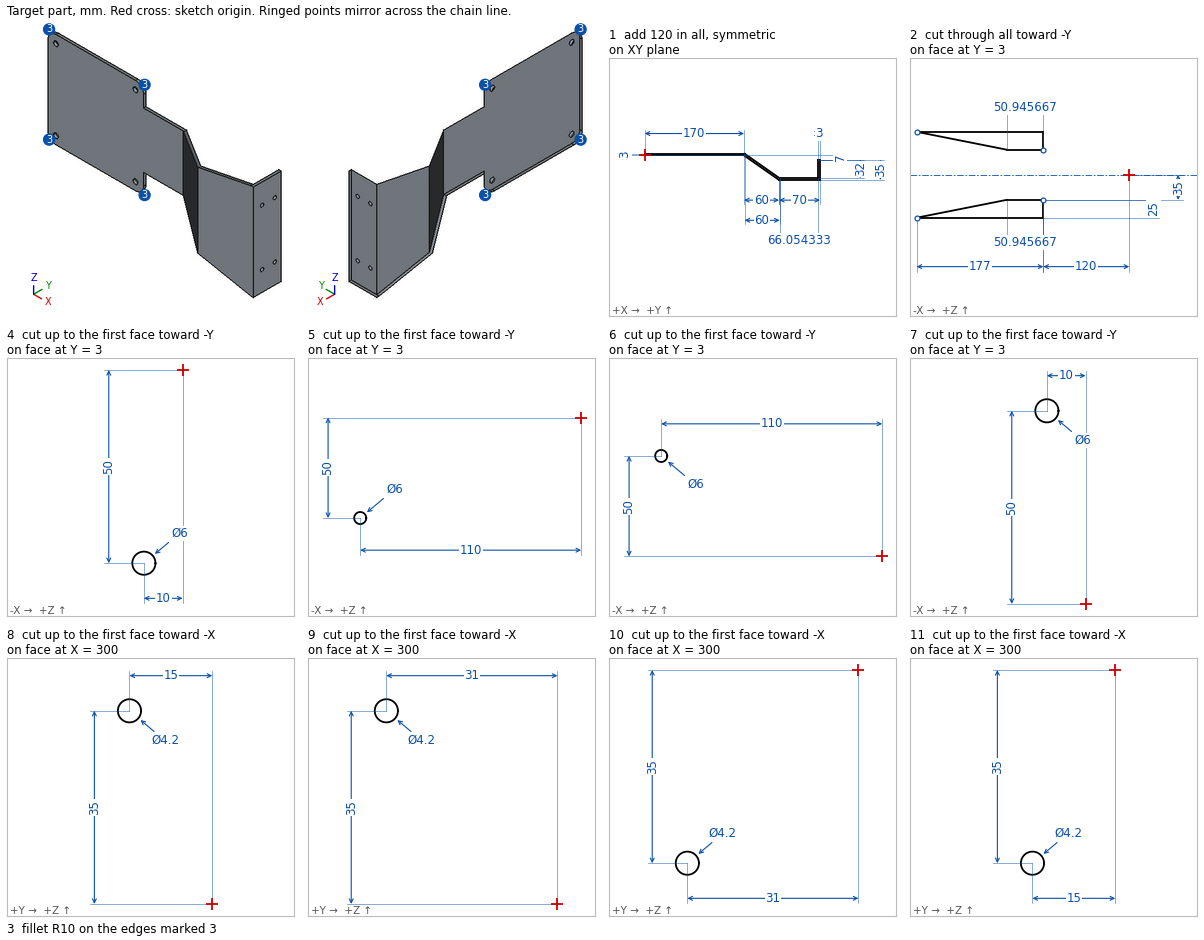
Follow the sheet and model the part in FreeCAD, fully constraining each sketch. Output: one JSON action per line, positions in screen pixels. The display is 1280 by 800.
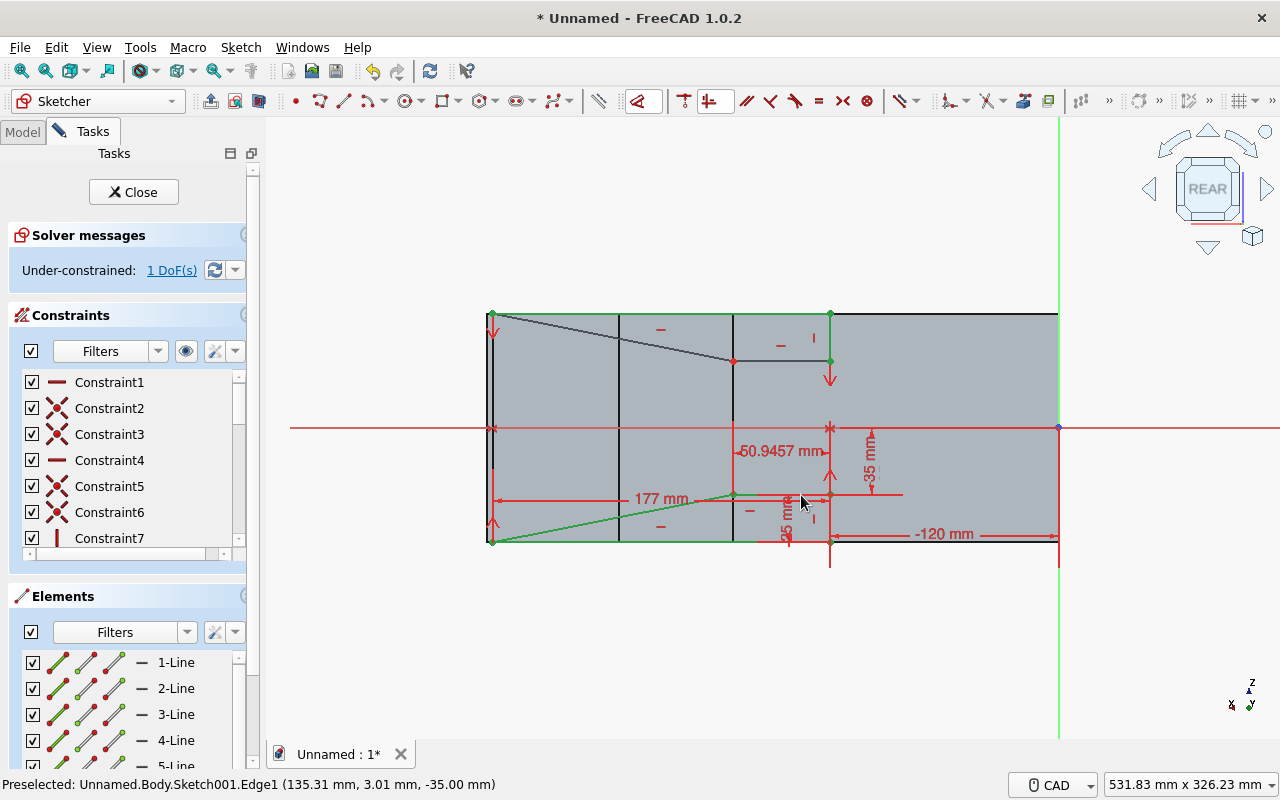
{"action": "left_click", "coordinate": [762, 361]}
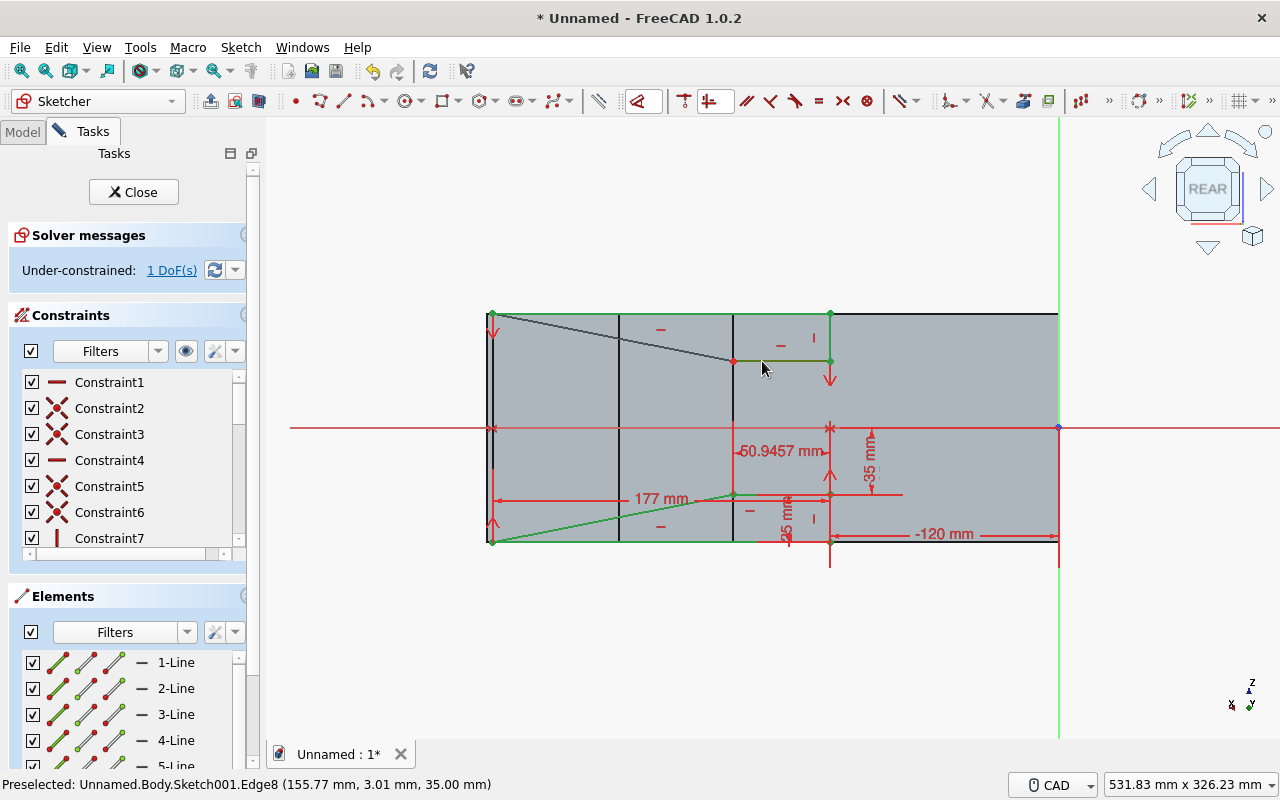
{"action": "key", "text": "l"}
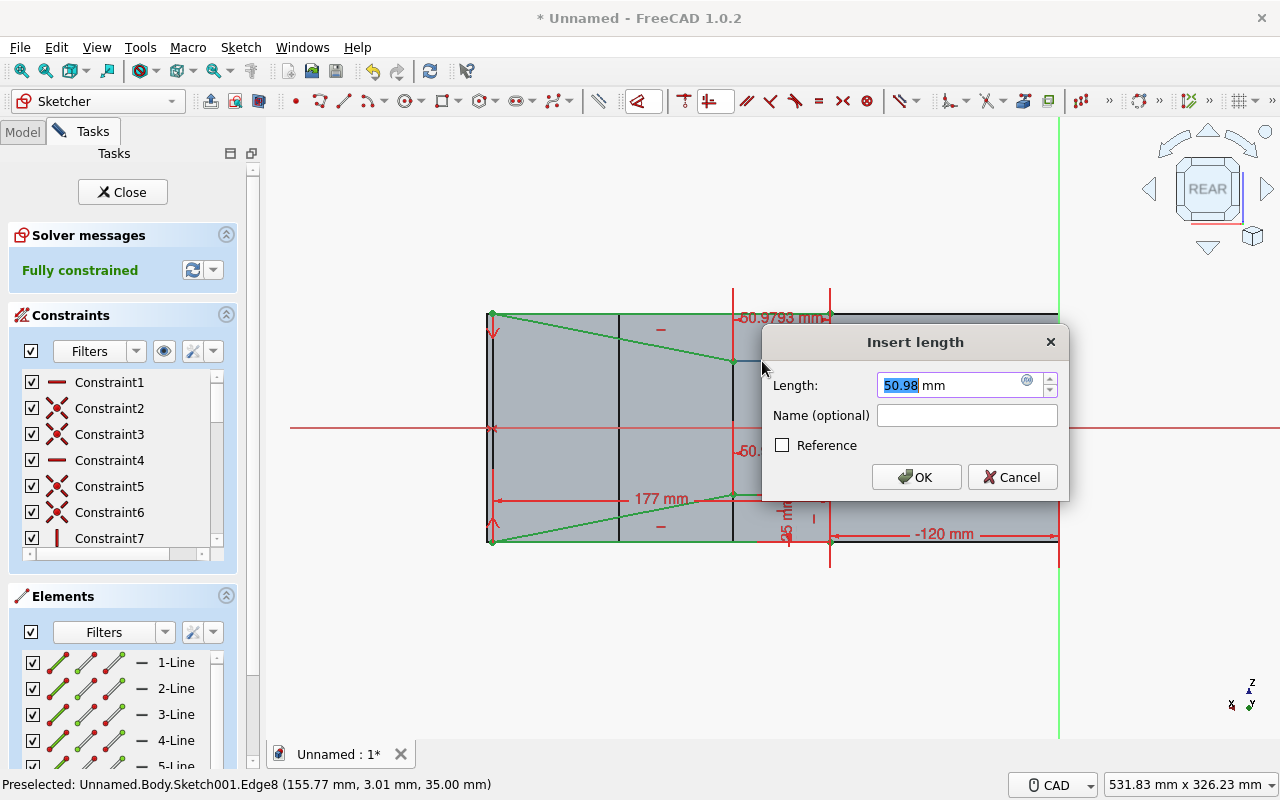
{"action": "type", "text": "50.945667"}
{"action": "key", "text": "Return"}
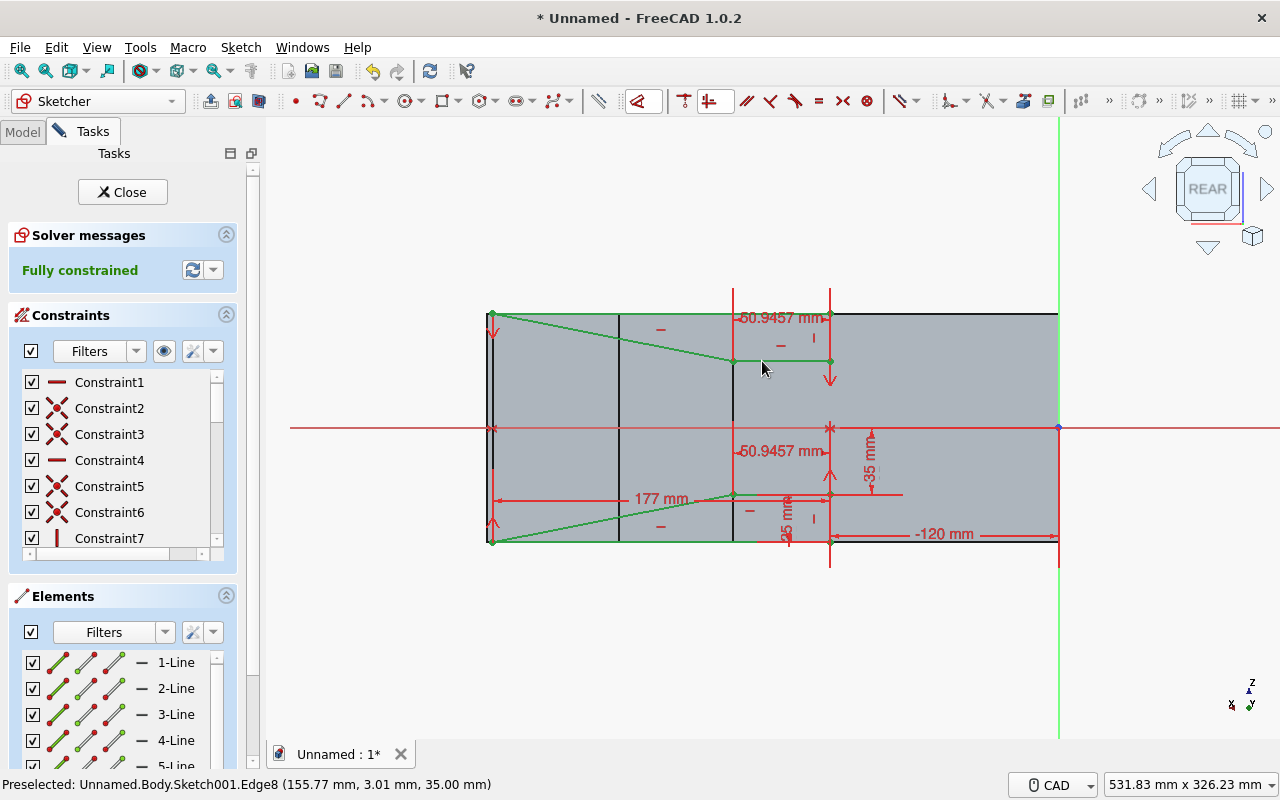
{"action": "left_click", "coordinate": [123, 192]}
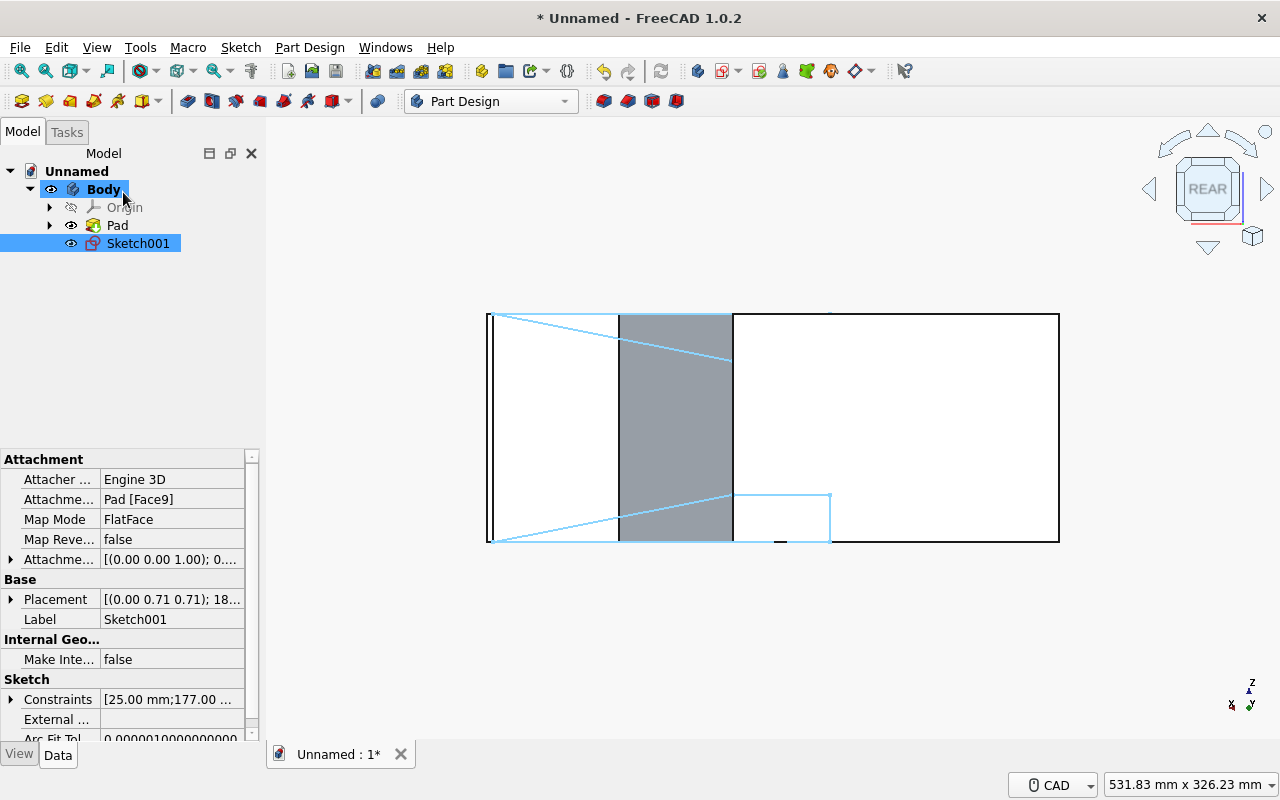
{"action": "left_click", "coordinate": [188, 102]}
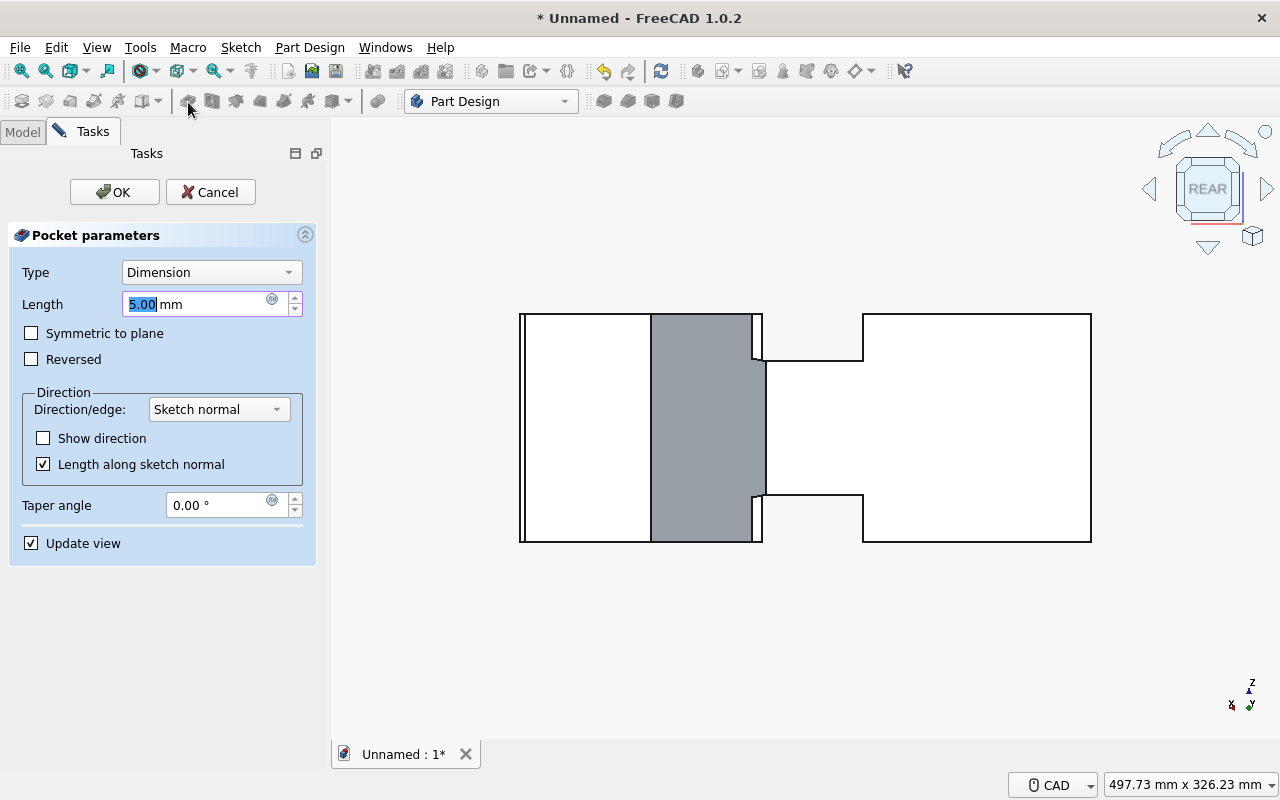
{"action": "left_click", "coordinate": [212, 272]}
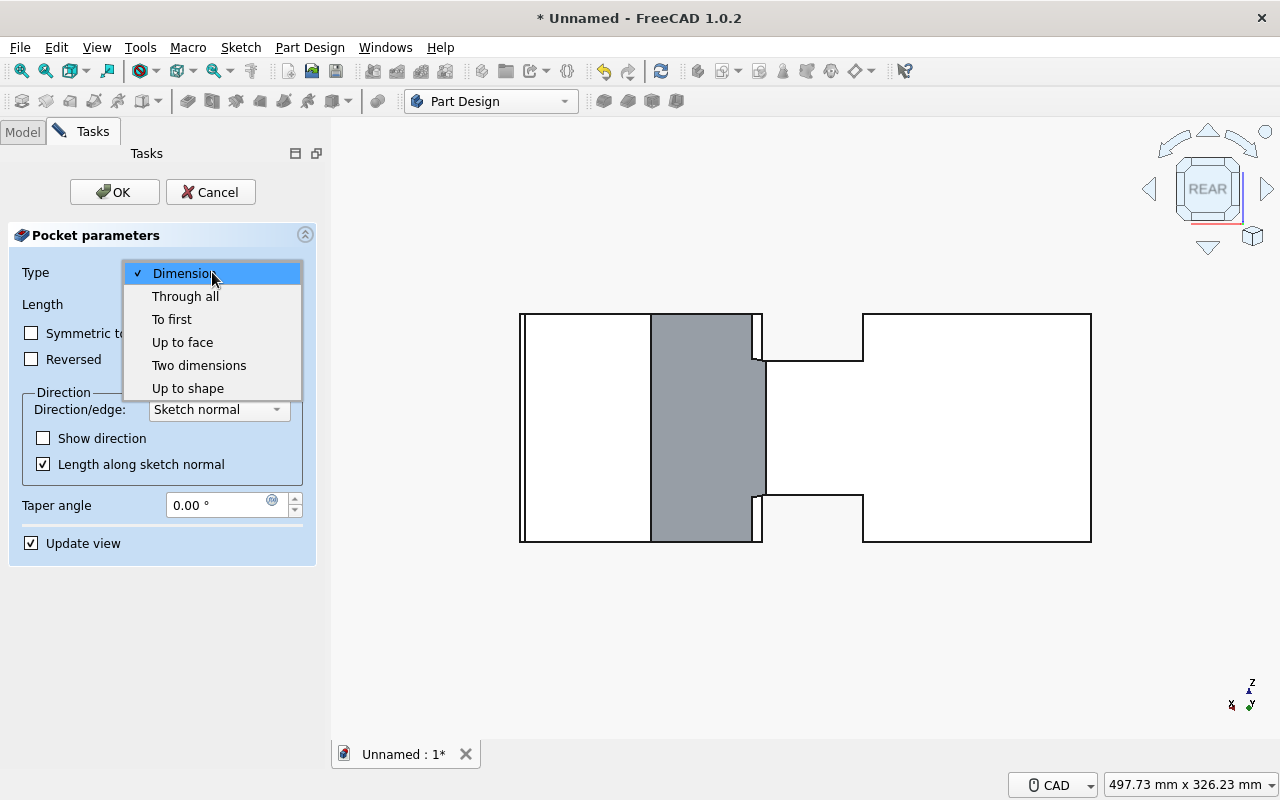
{"action": "left_click", "coordinate": [212, 296]}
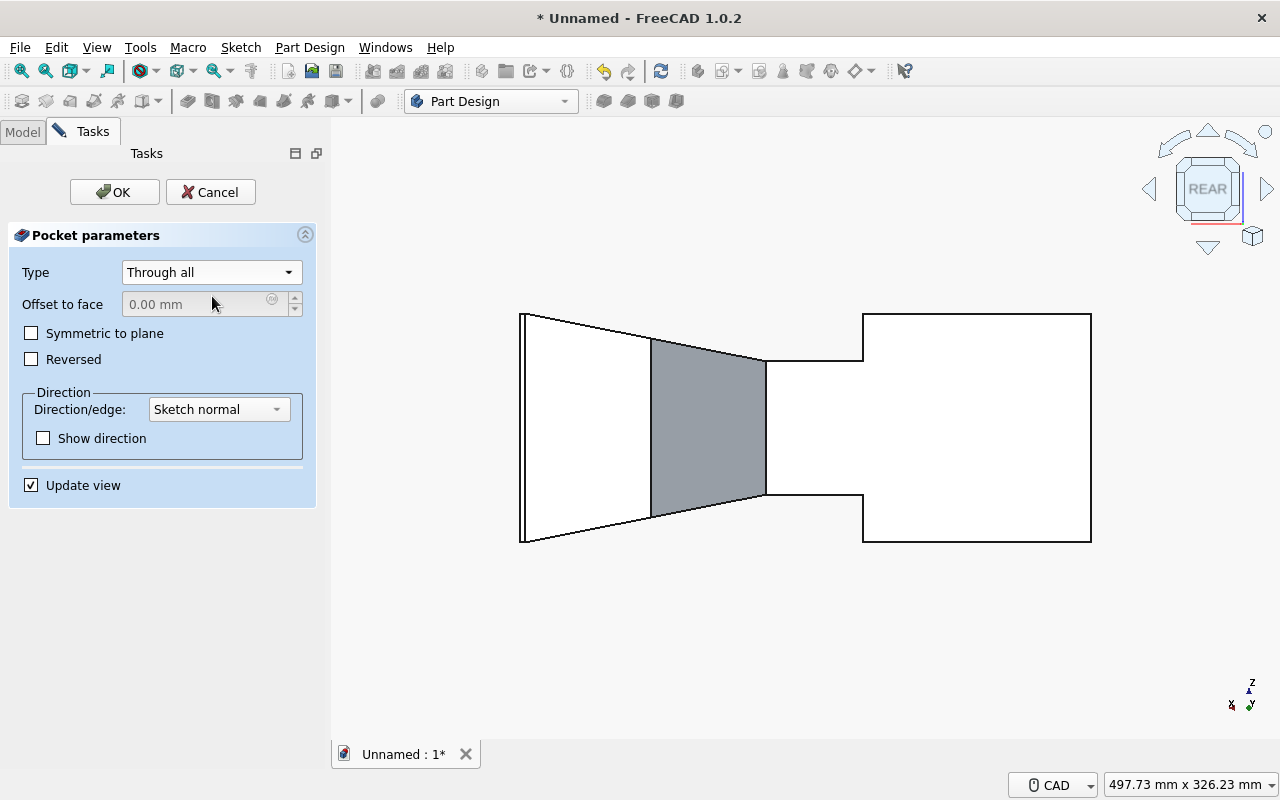
{"action": "left_click", "coordinate": [115, 192]}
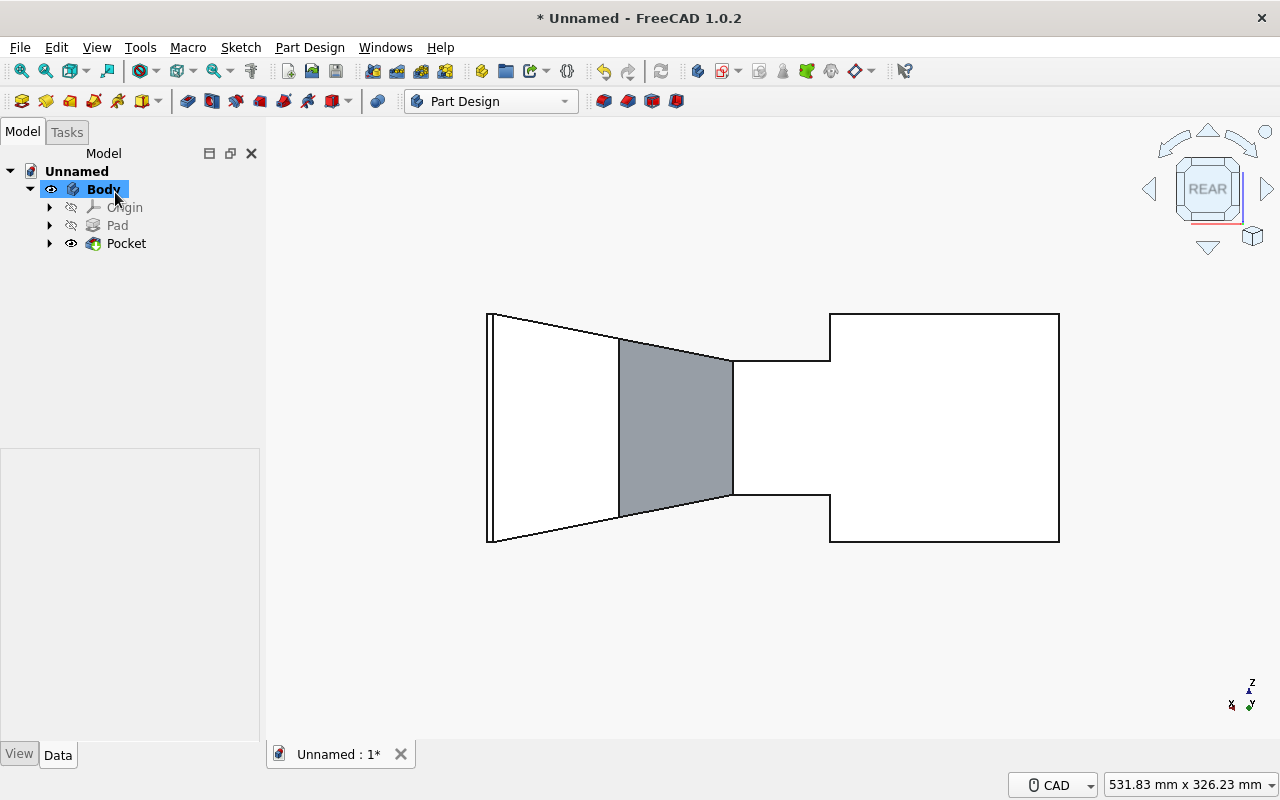
{"action": "scroll", "coordinate": [1059, 541], "scroll_direction": "up", "scroll_amount": 10}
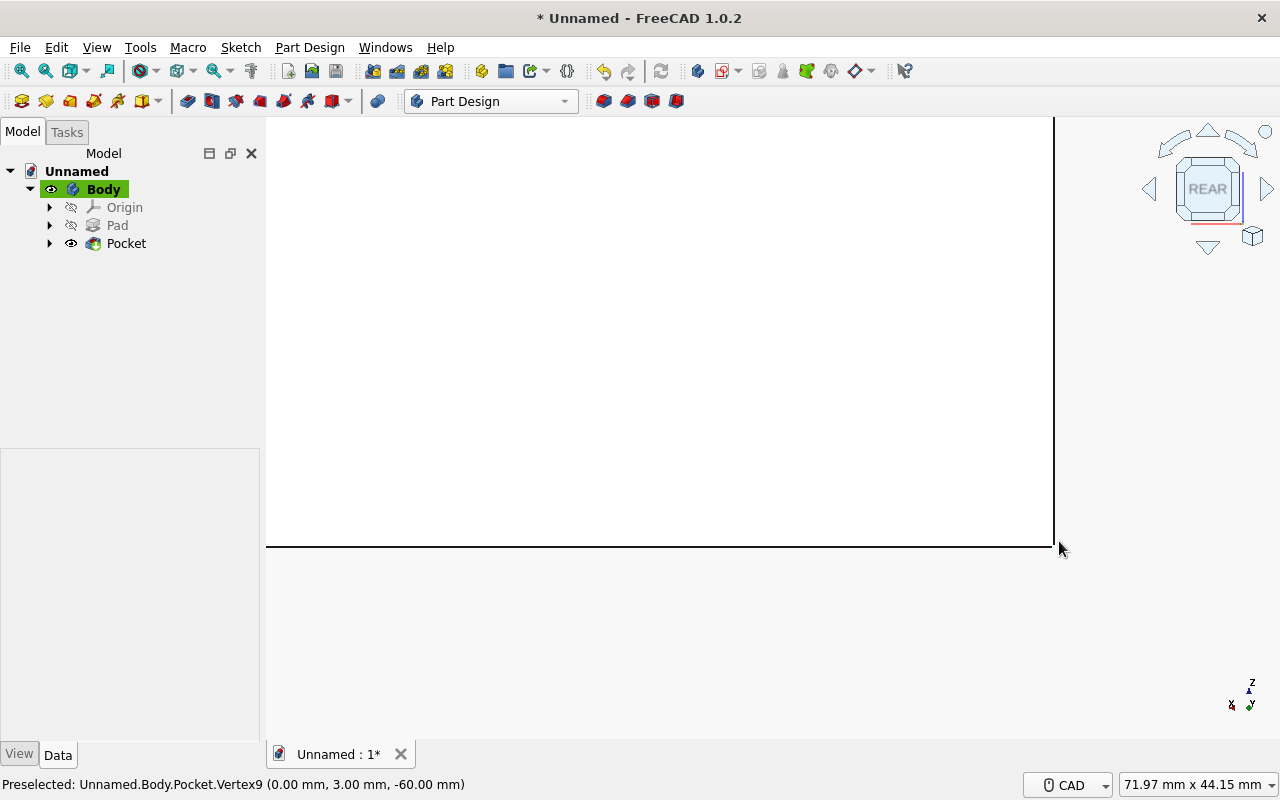
{"action": "left_click", "coordinate": [22, 72]}